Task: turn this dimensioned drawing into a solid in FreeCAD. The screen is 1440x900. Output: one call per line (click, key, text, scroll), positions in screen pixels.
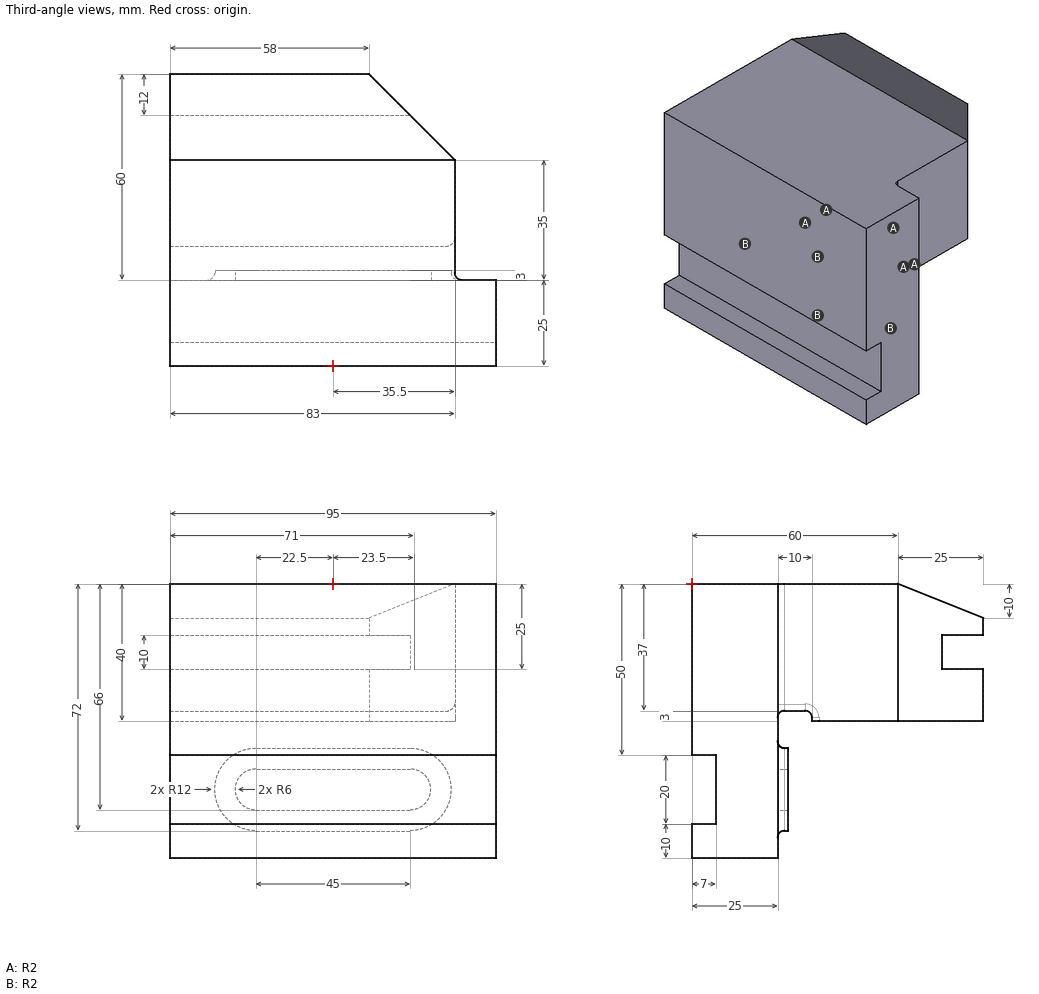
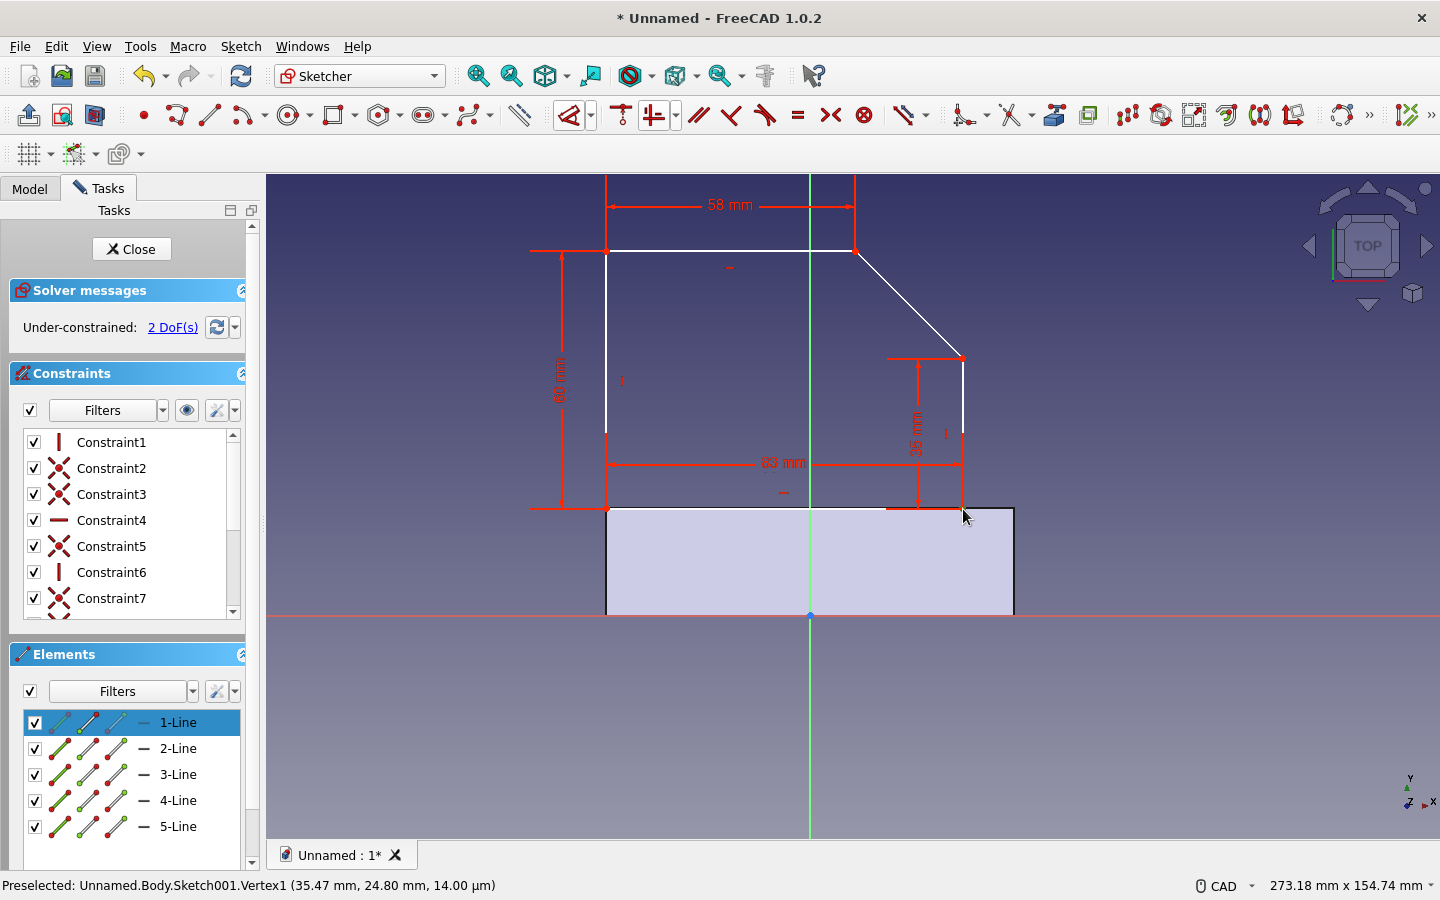
click(590, 116)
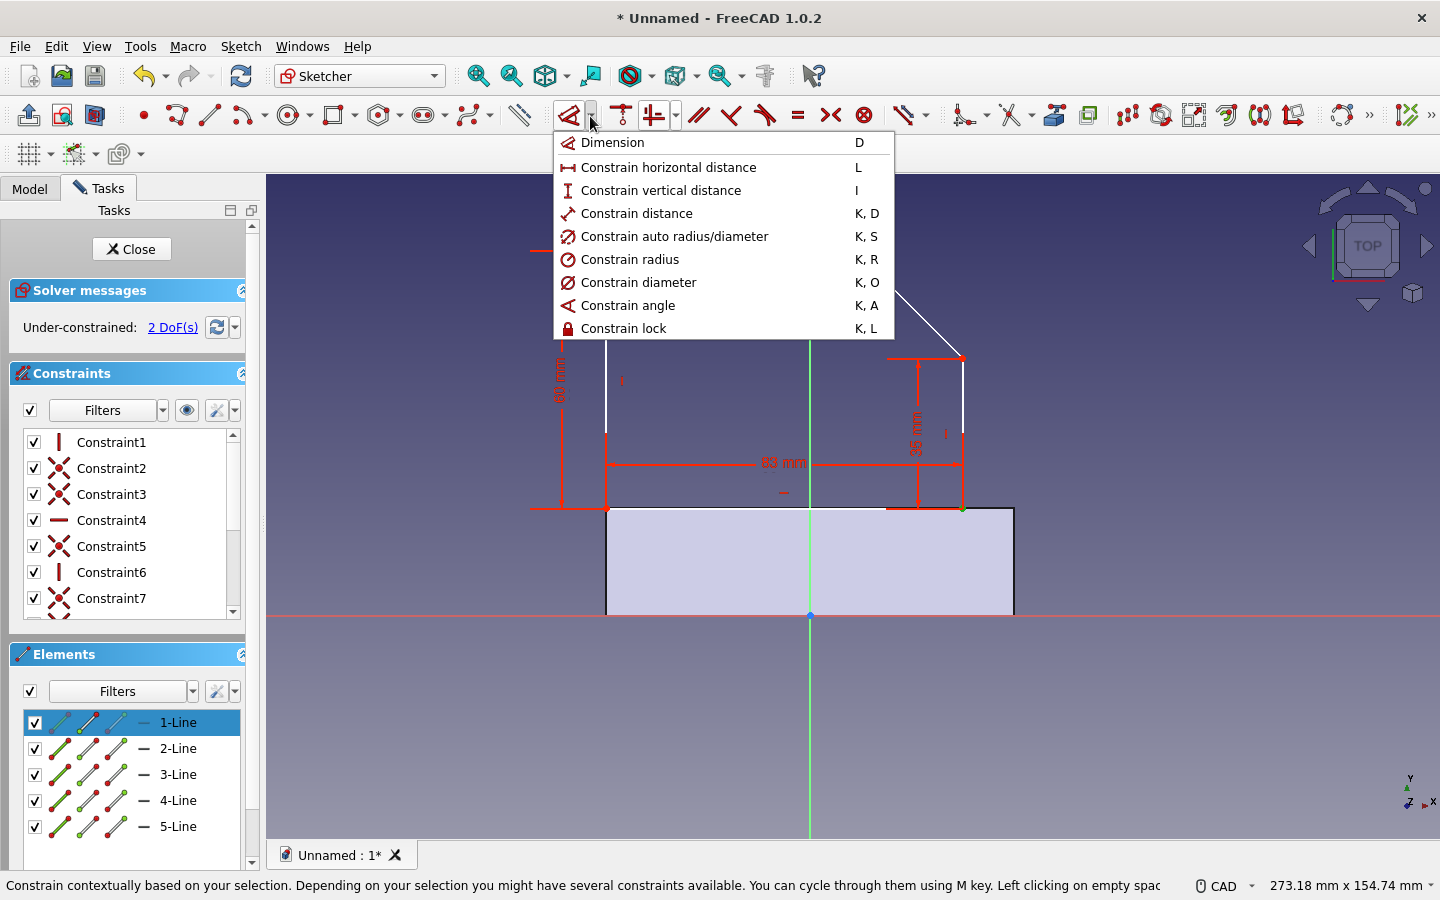
click(724, 190)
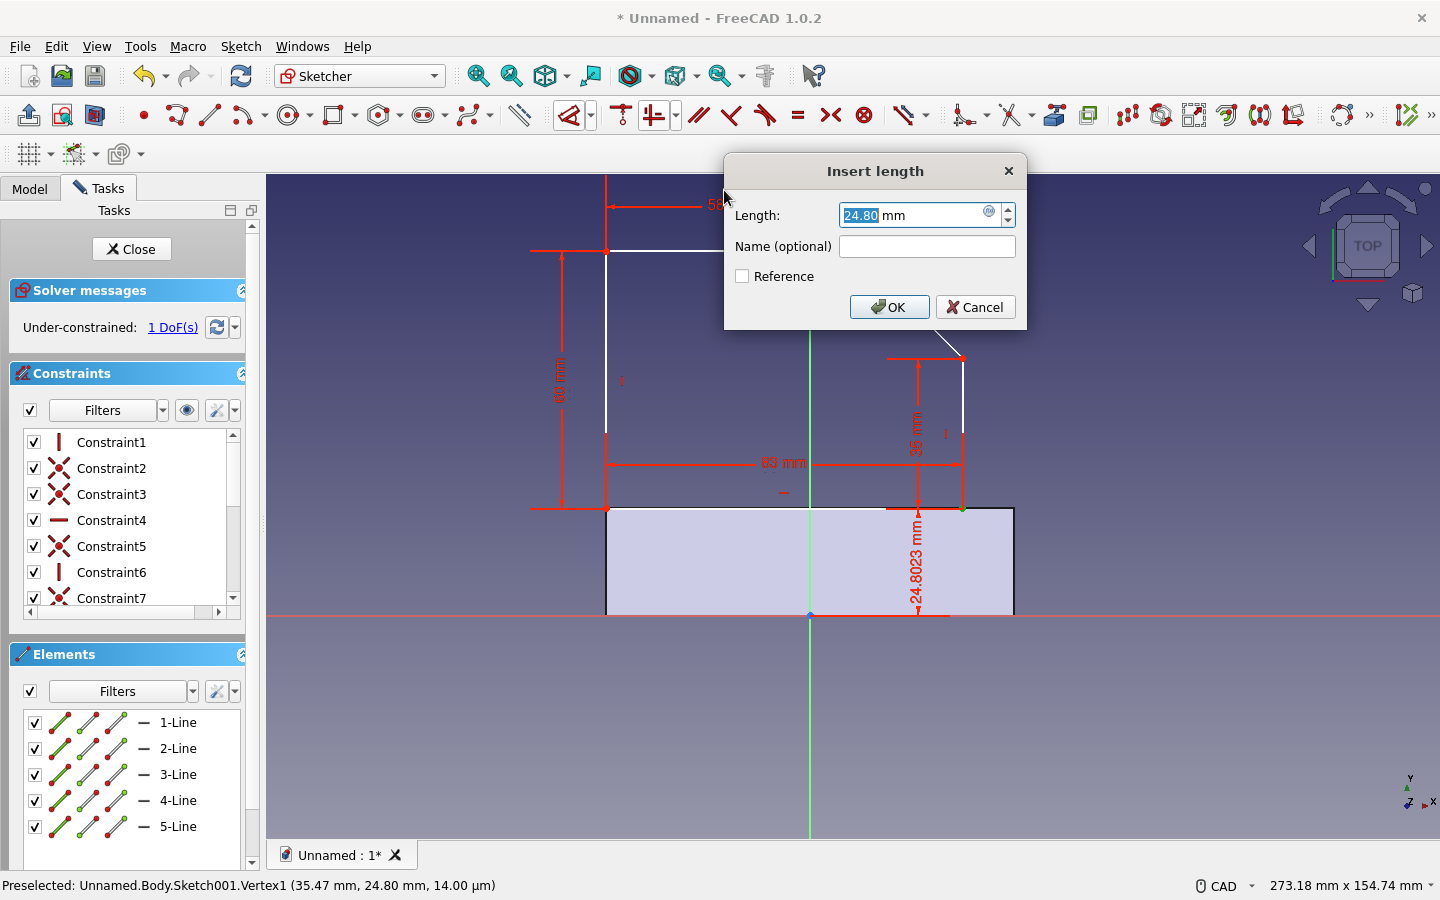
text(25)
key(Return)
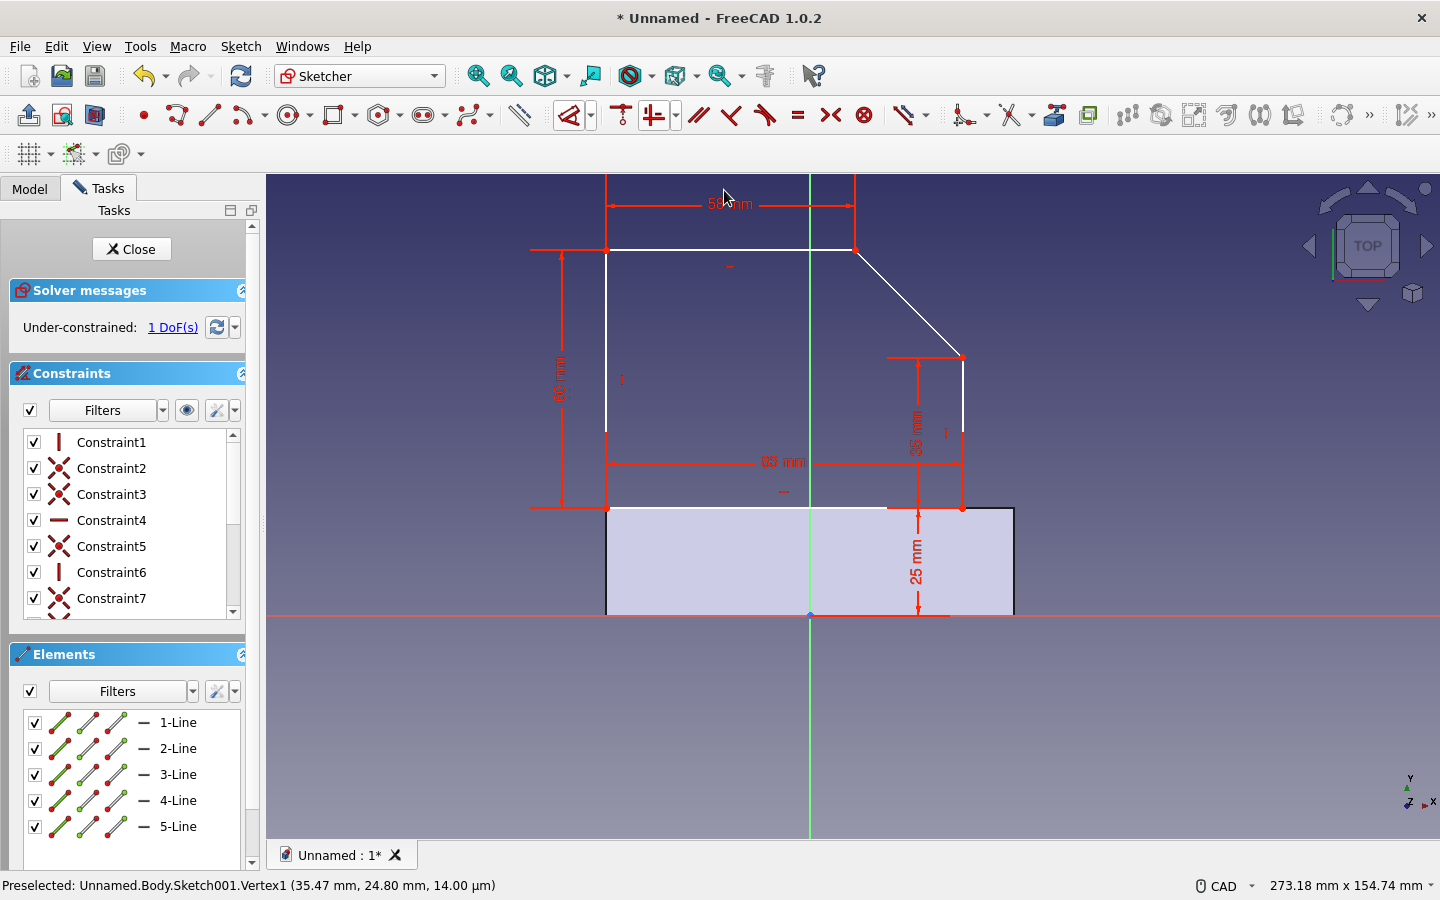
click(963, 508)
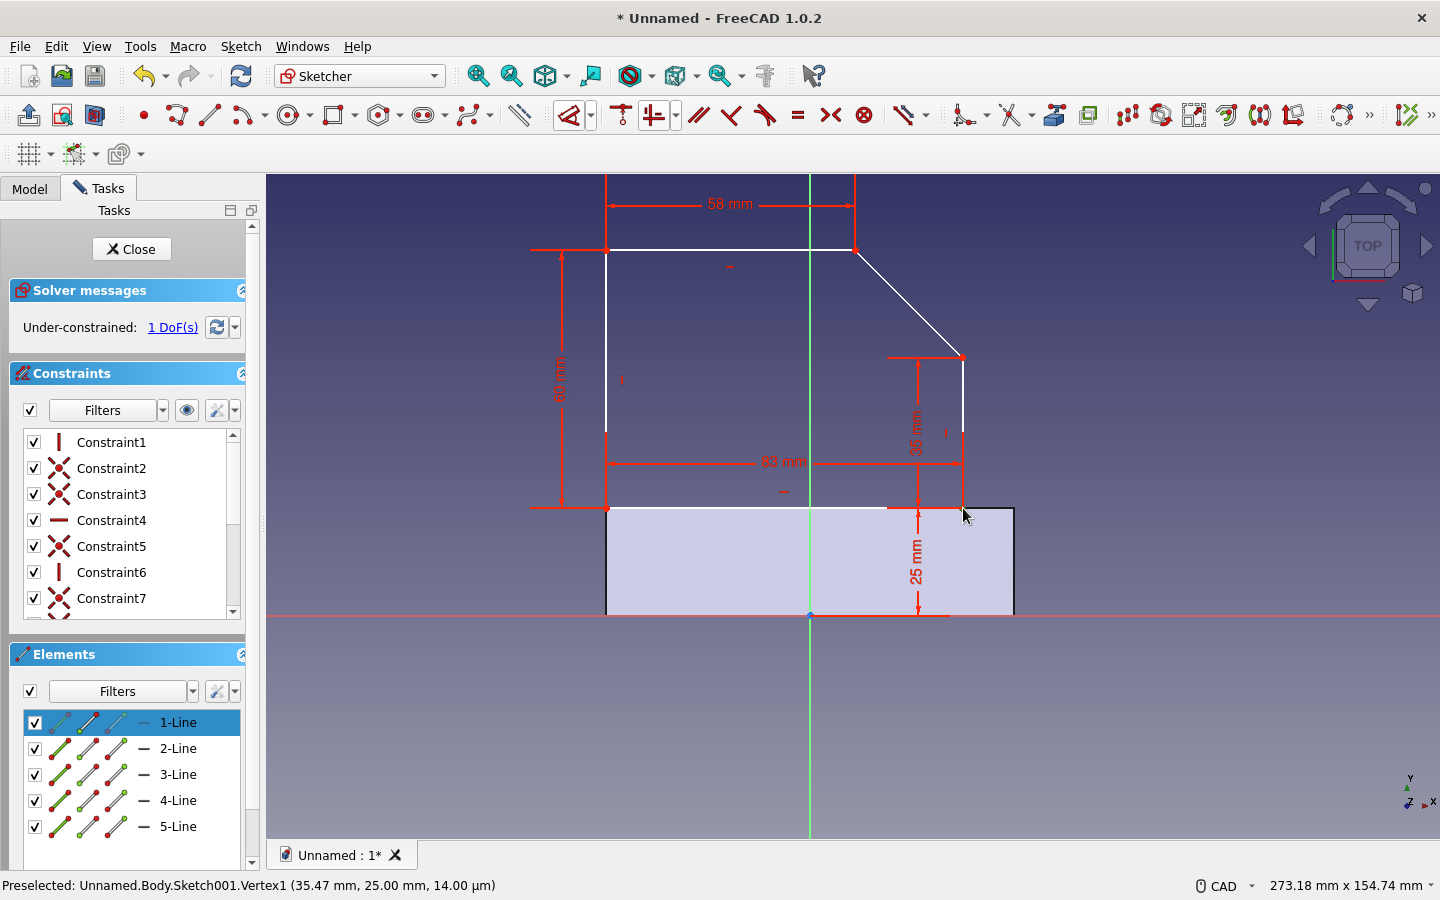
key(l)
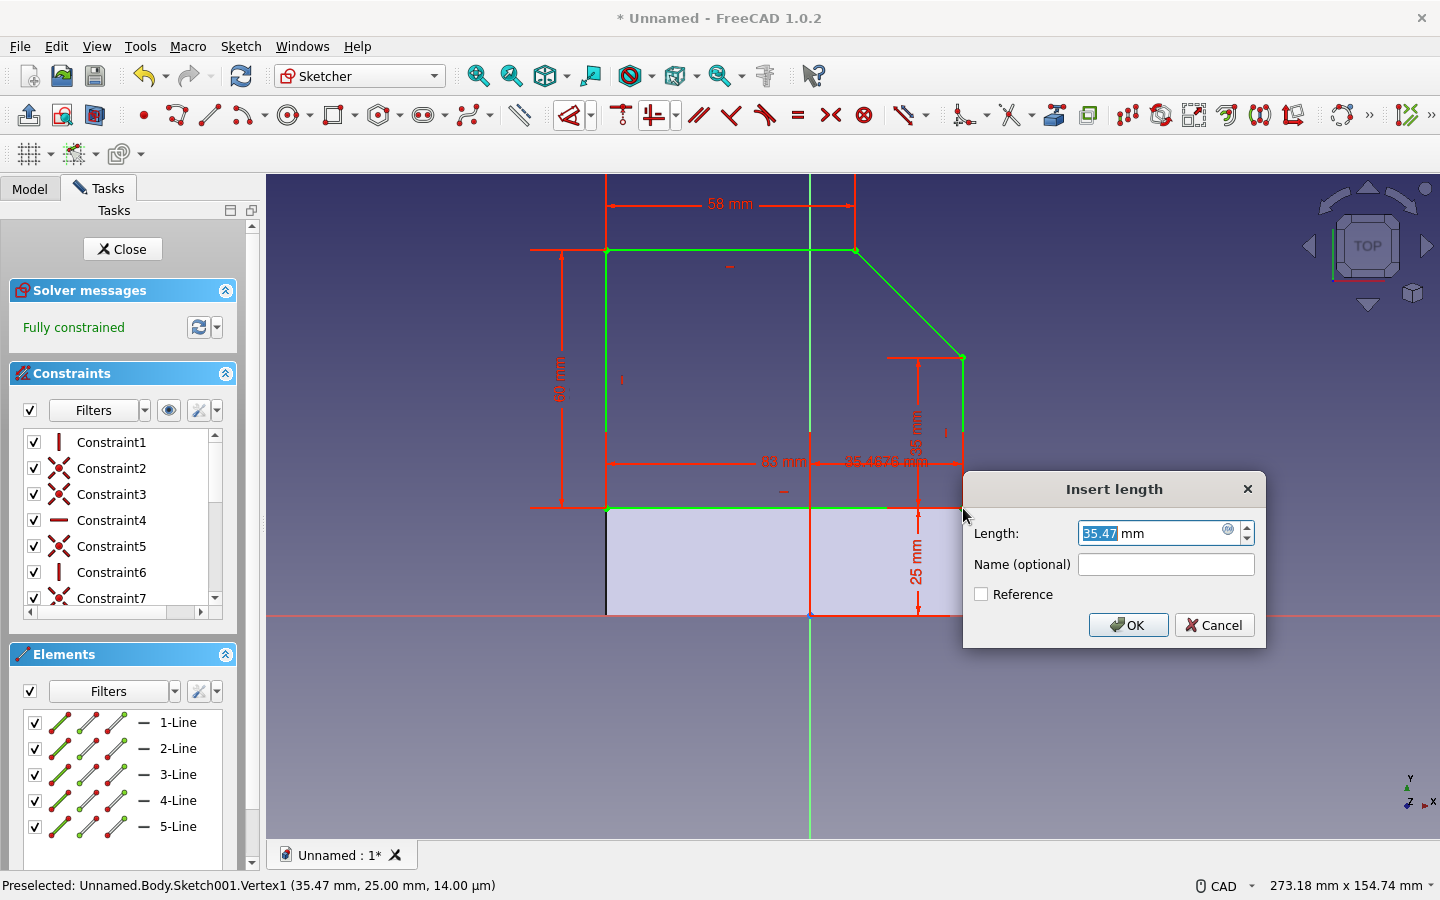
text(35.5)
key(Return)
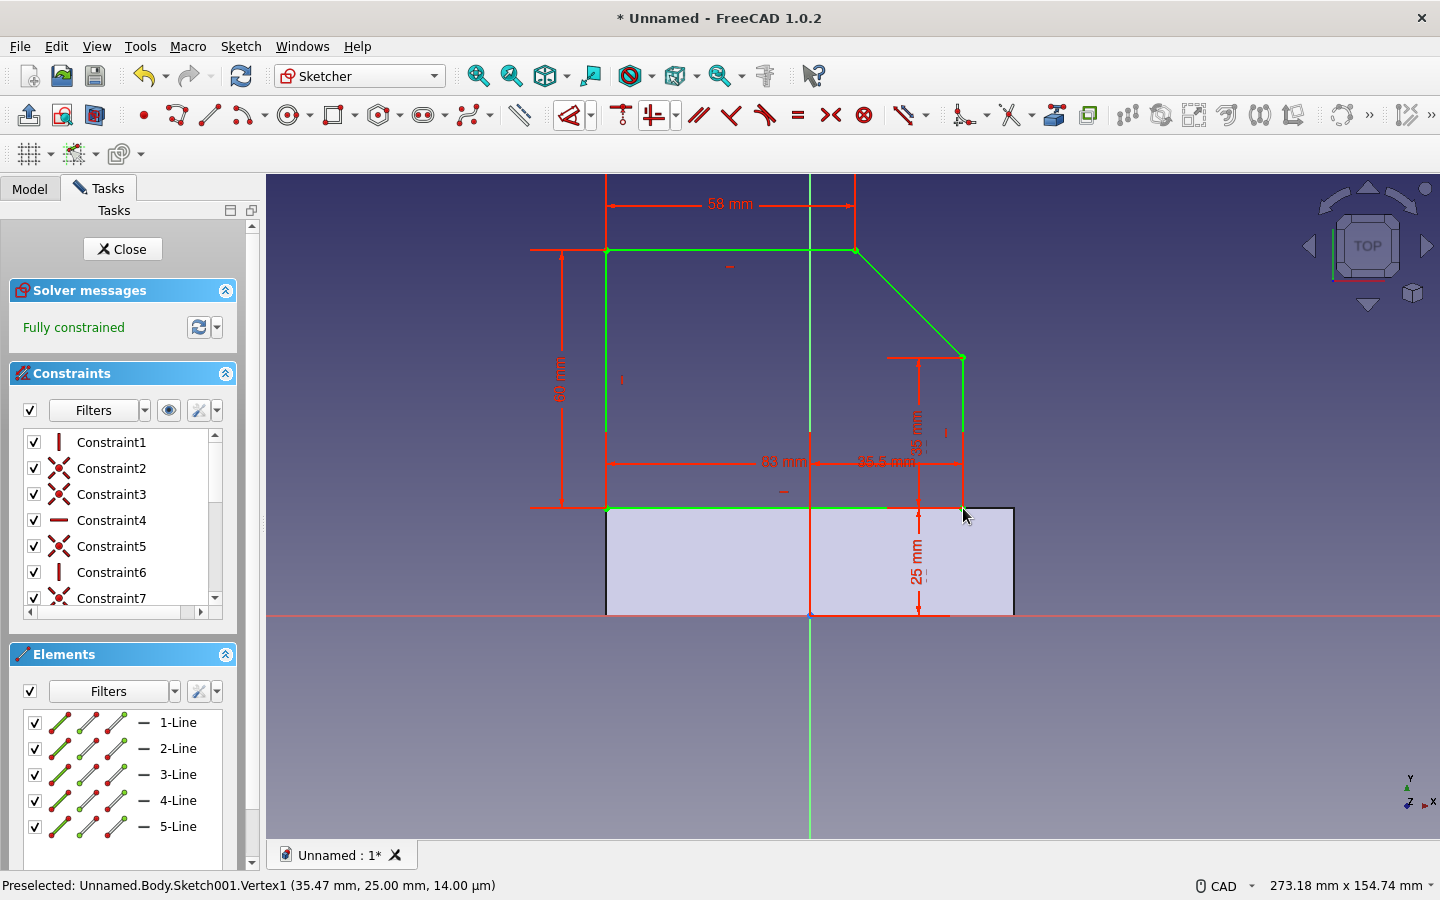
click(123, 249)